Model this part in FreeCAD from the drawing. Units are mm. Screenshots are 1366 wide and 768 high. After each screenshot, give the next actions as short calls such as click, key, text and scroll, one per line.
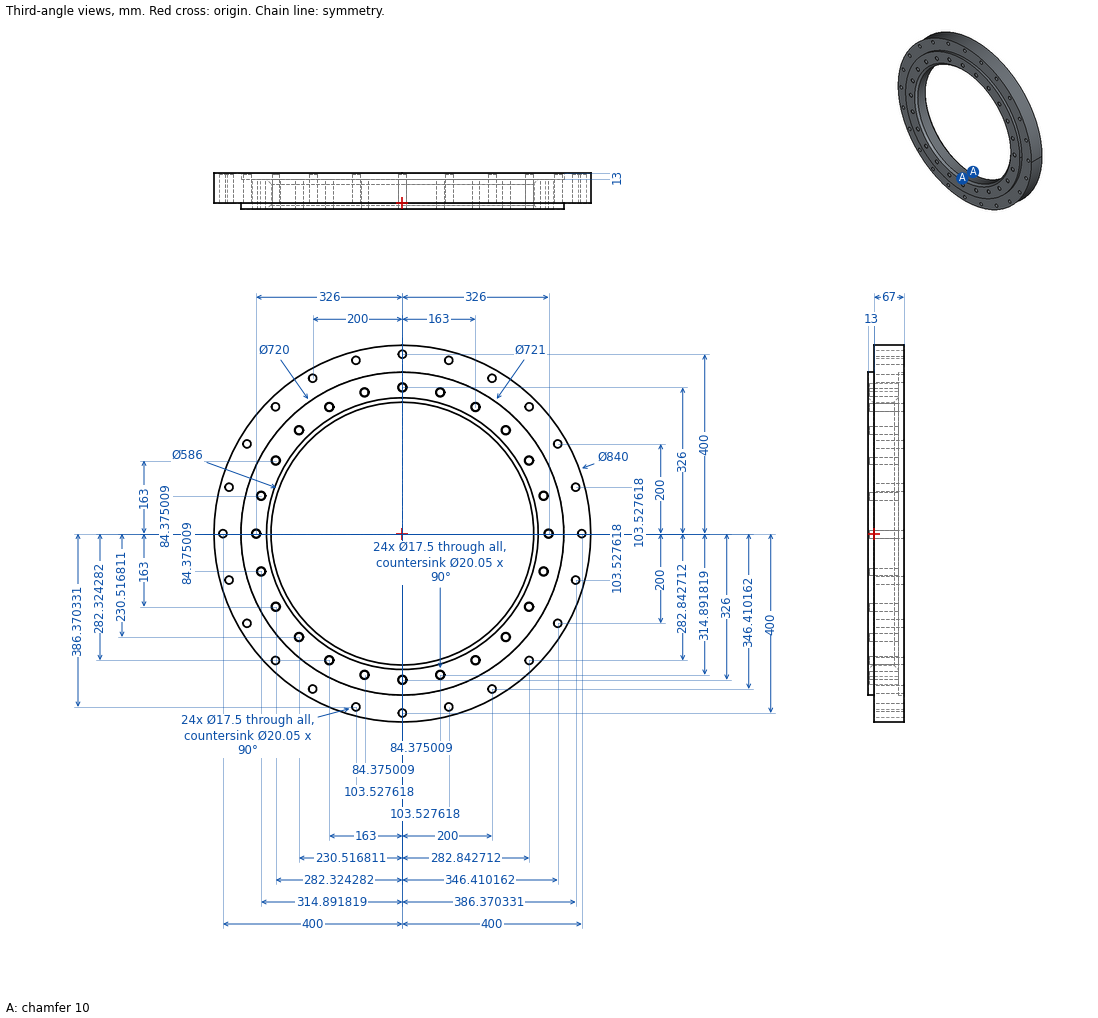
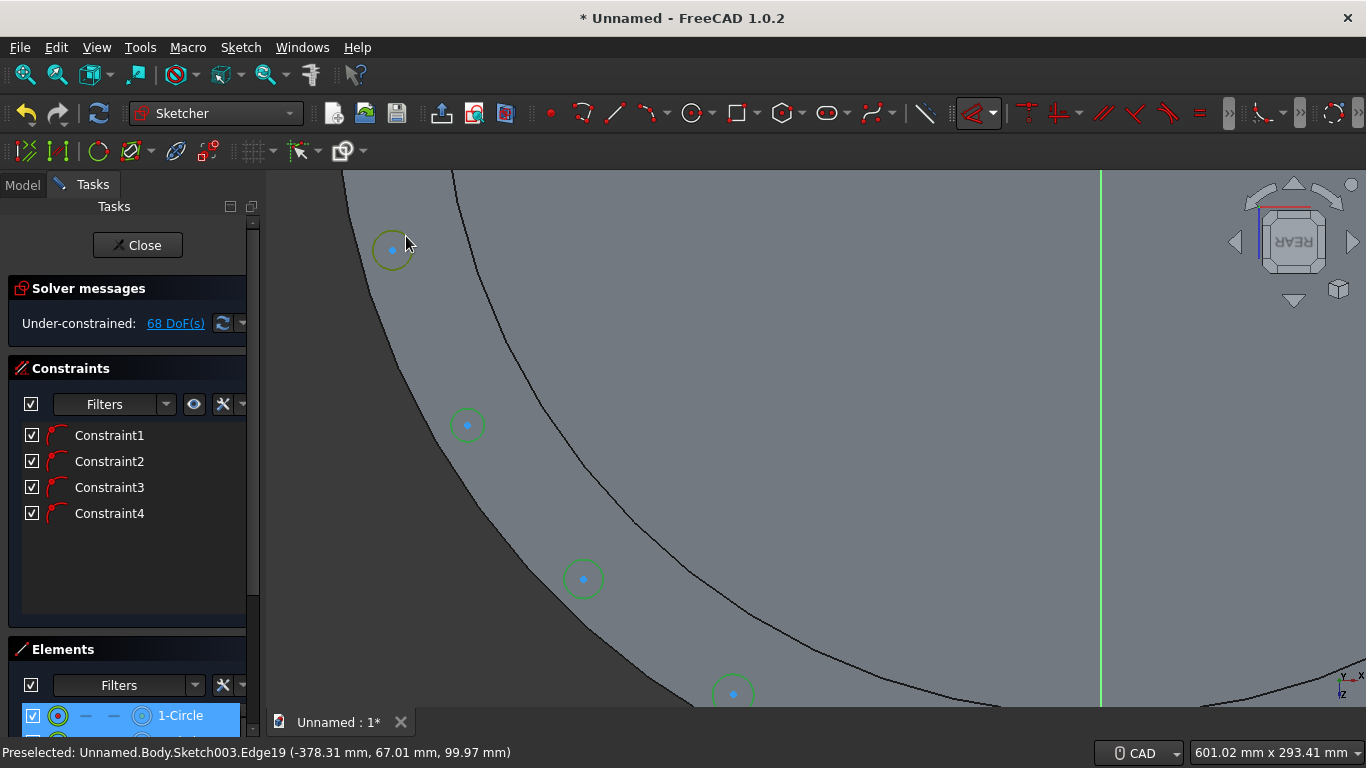
scroll(632, 564, down, 7)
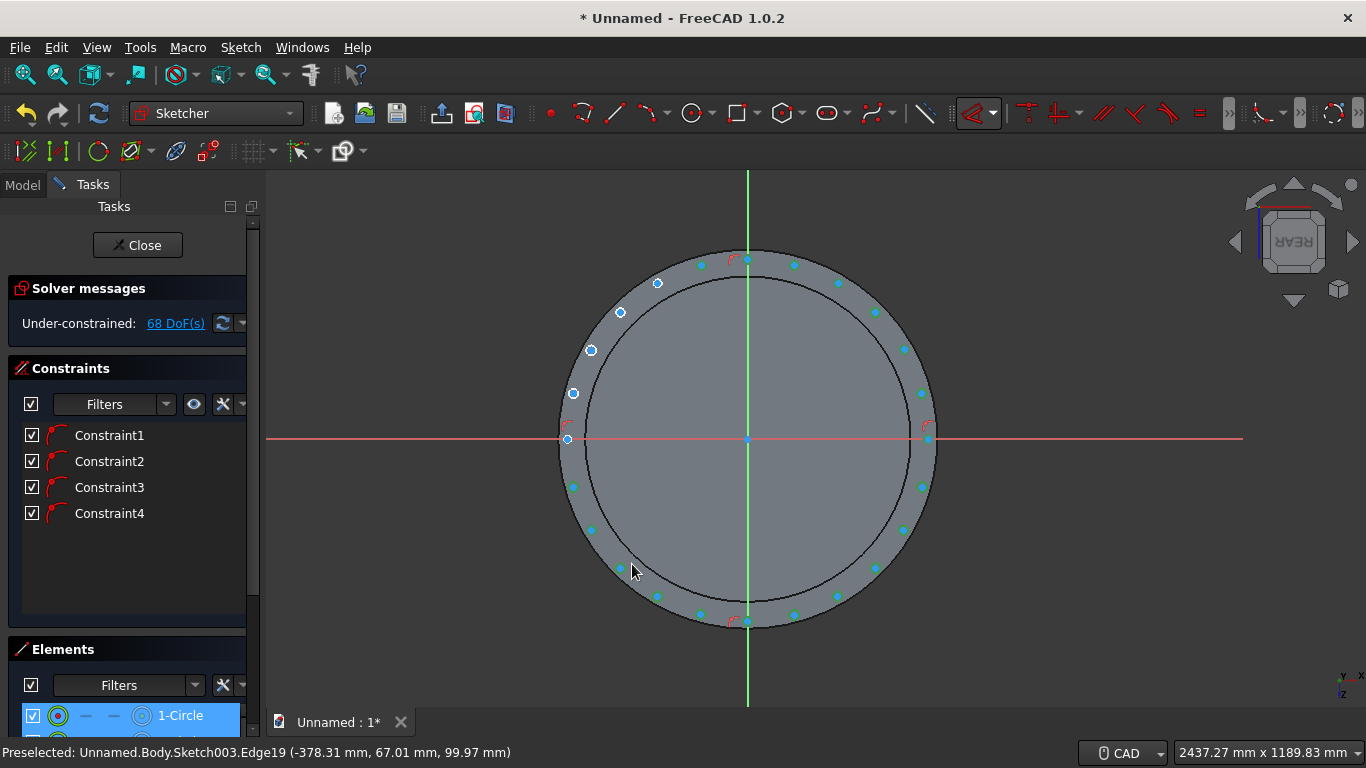
scroll(570, 437, up, 9)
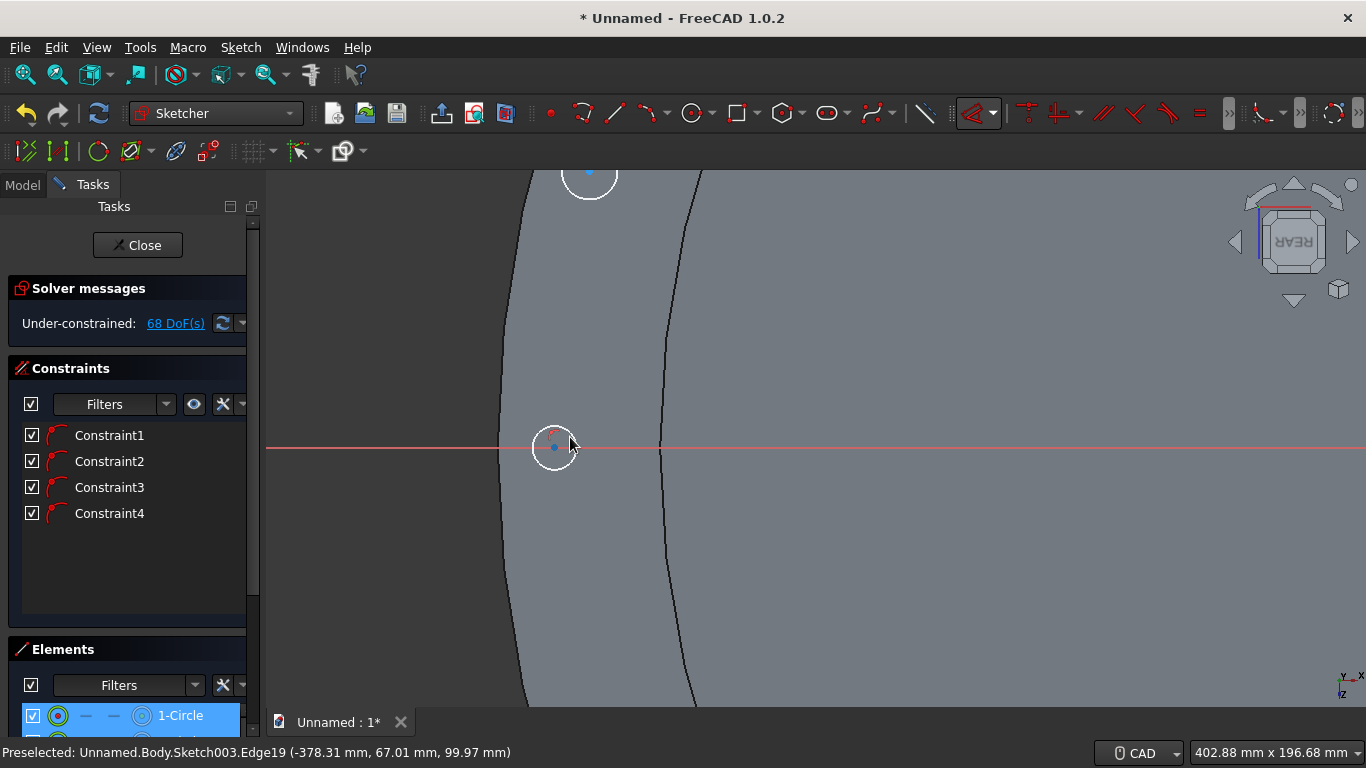
click(570, 432)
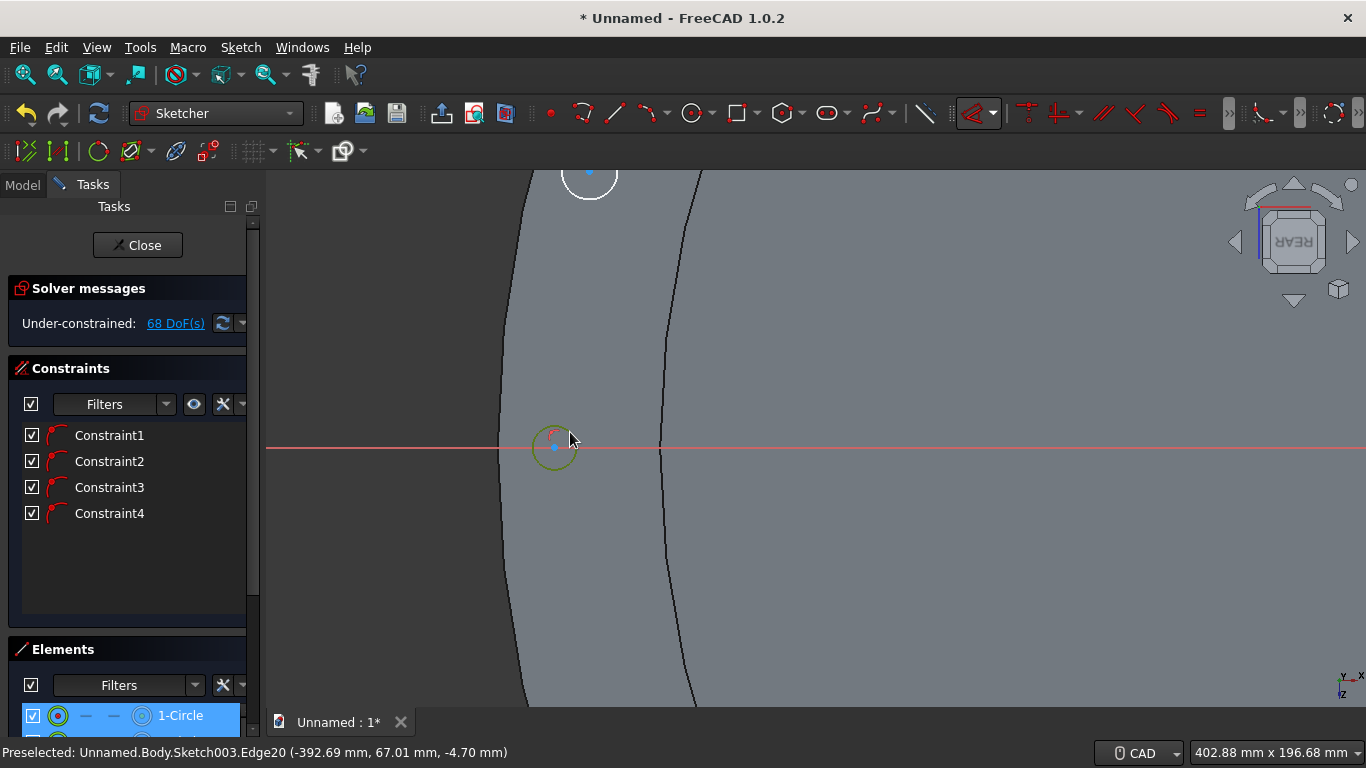
click(589, 199)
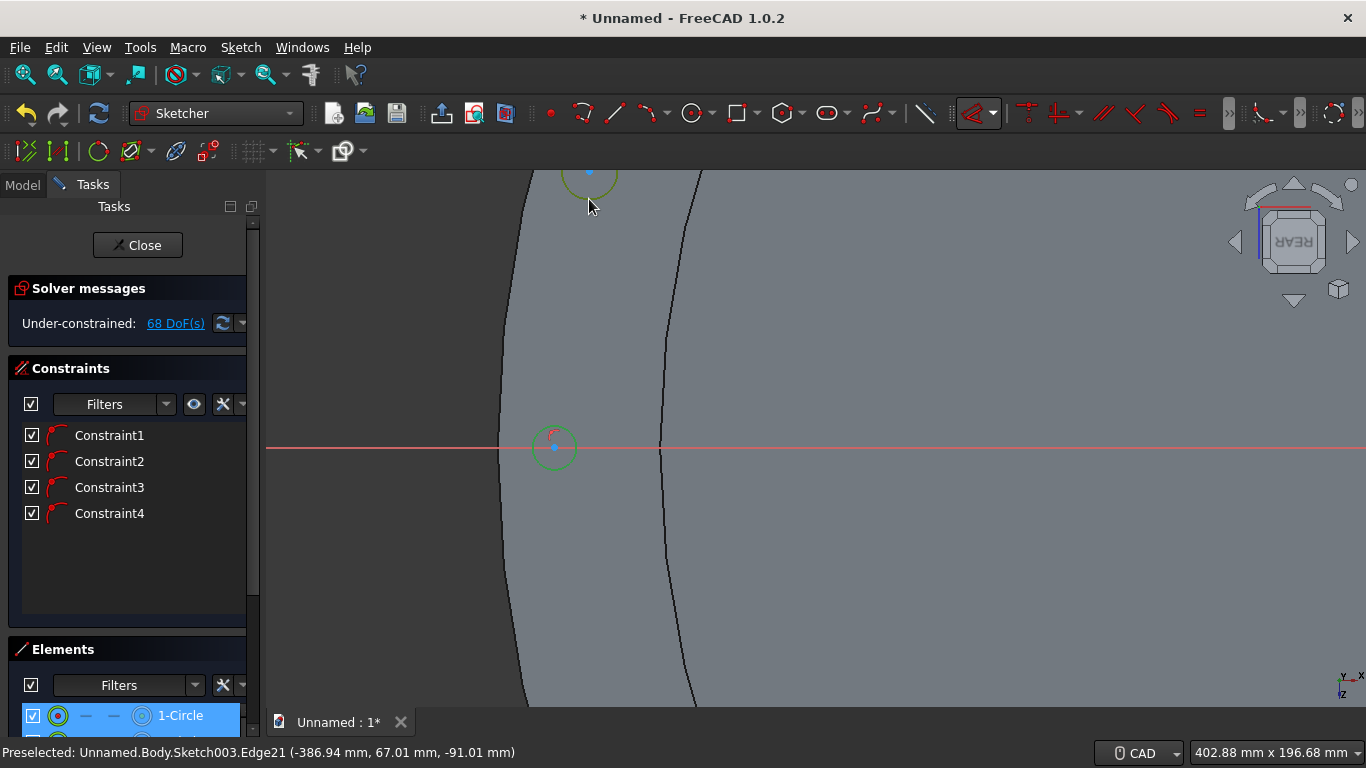
scroll(570, 437, down, 9)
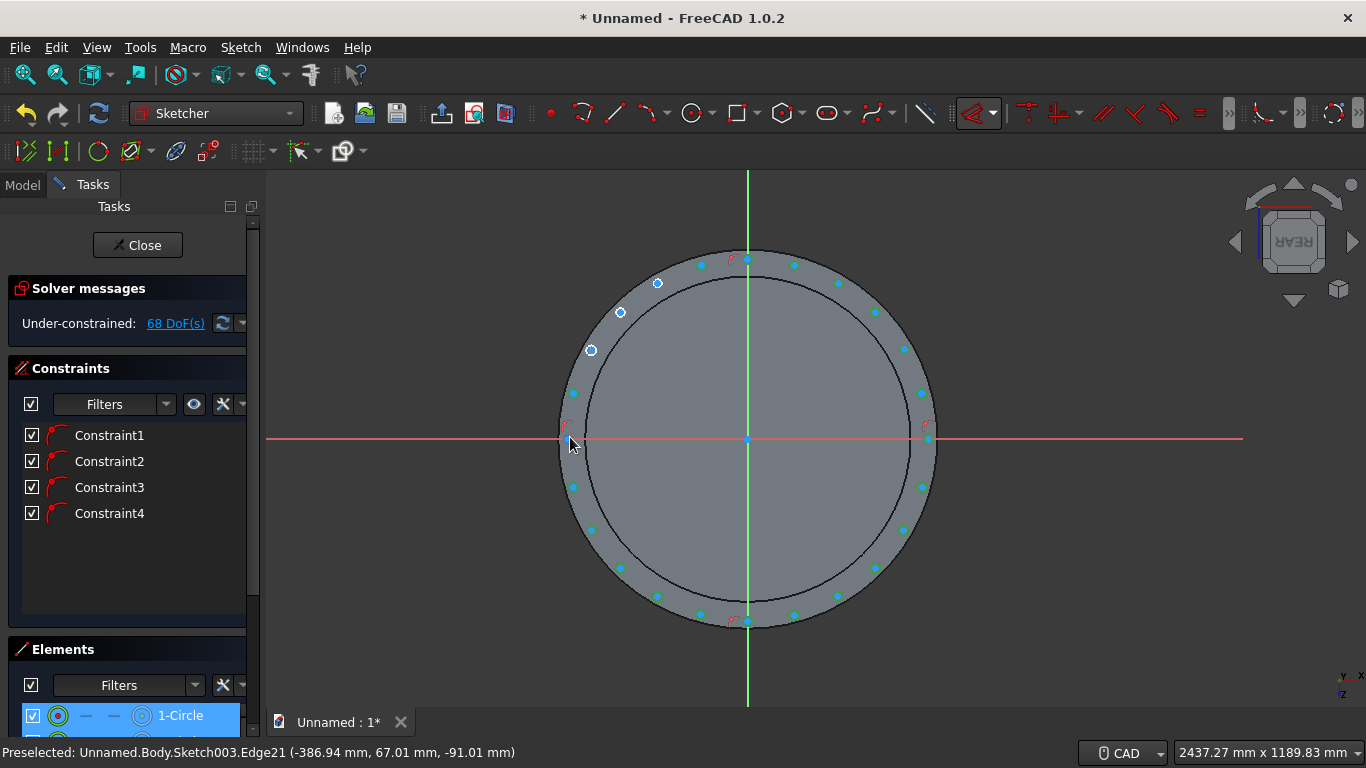
scroll(595, 347, up, 6)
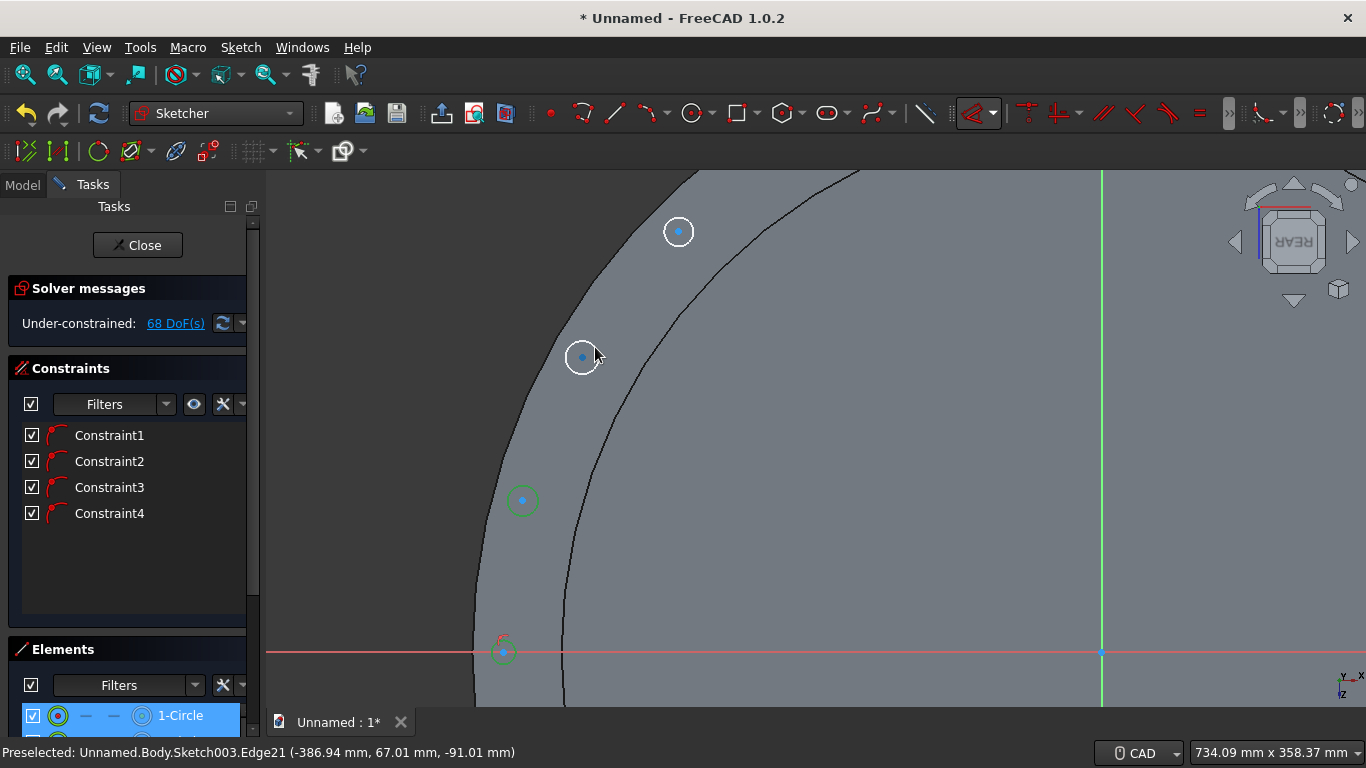
click(594, 346)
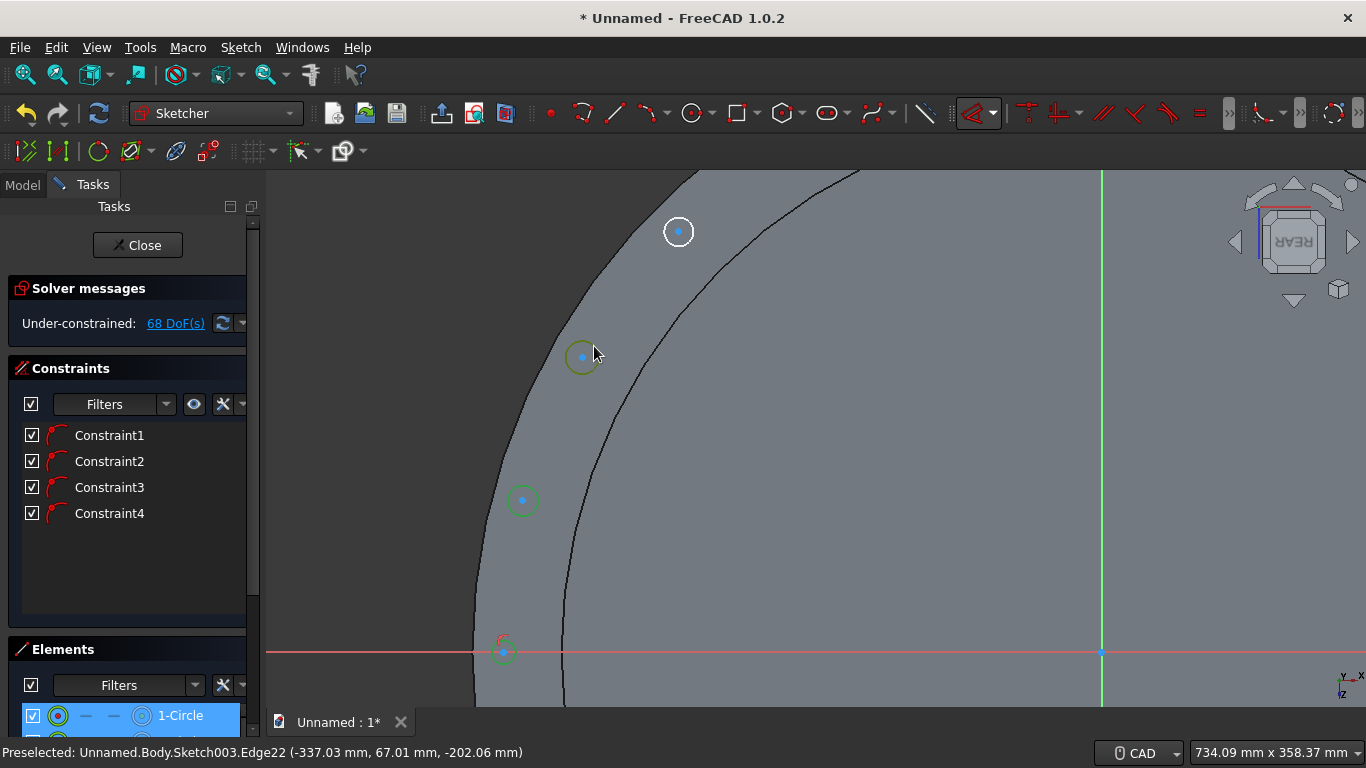
click(689, 222)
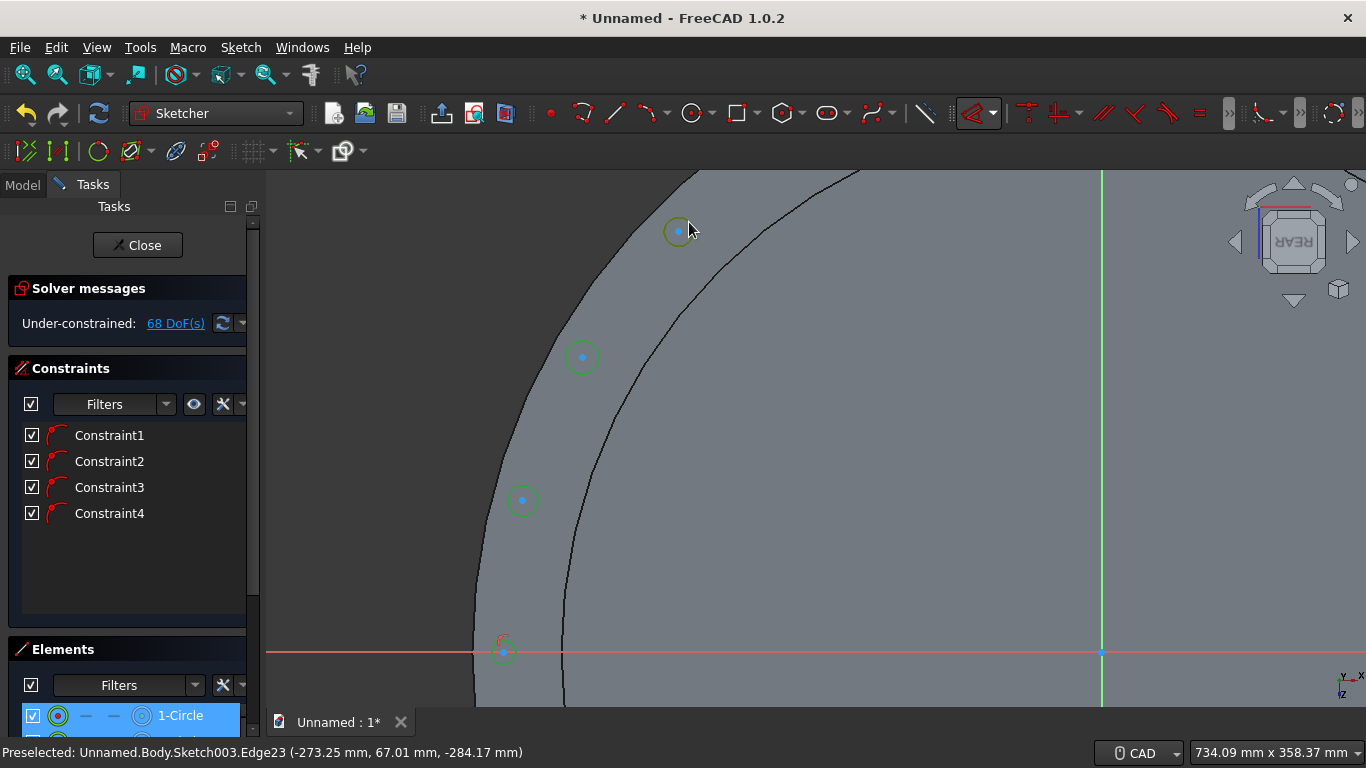
scroll(595, 346, down, 6)